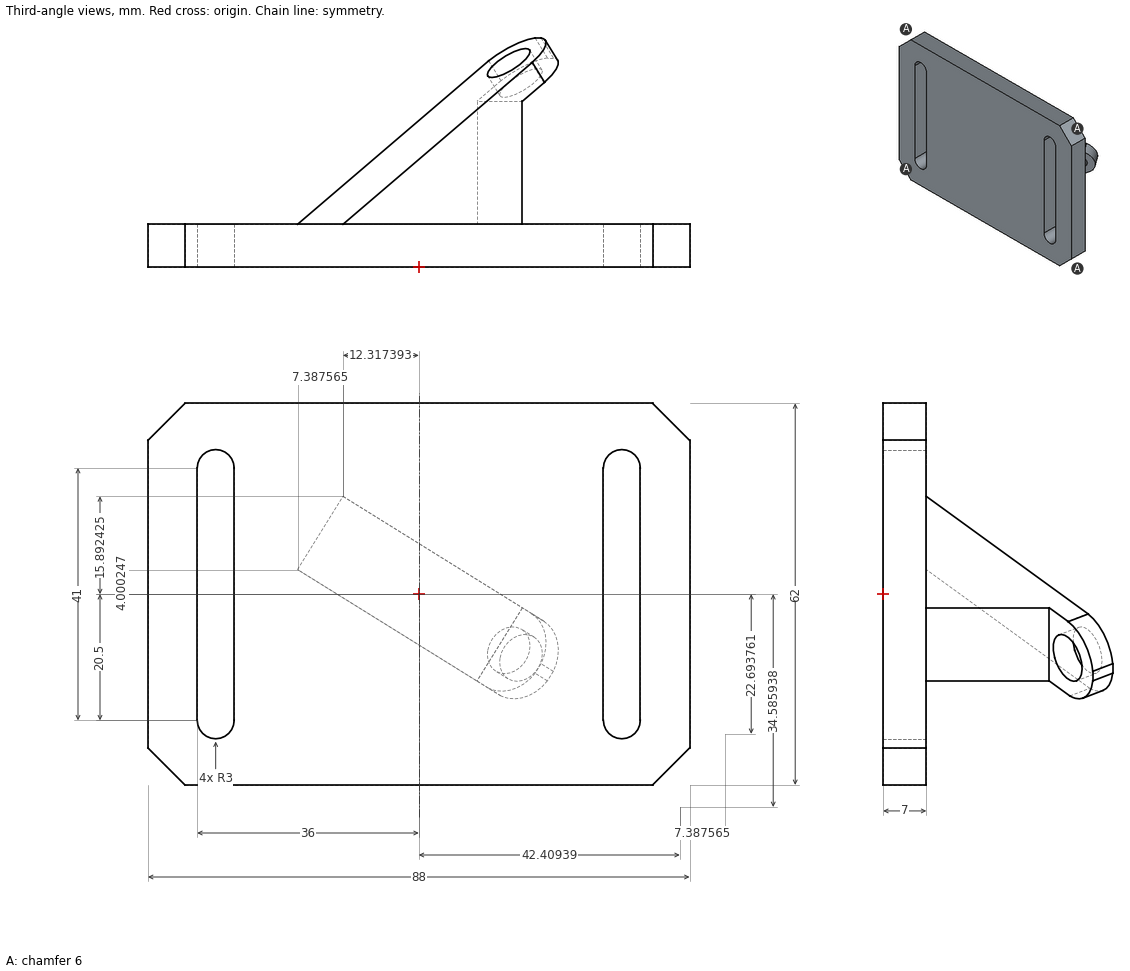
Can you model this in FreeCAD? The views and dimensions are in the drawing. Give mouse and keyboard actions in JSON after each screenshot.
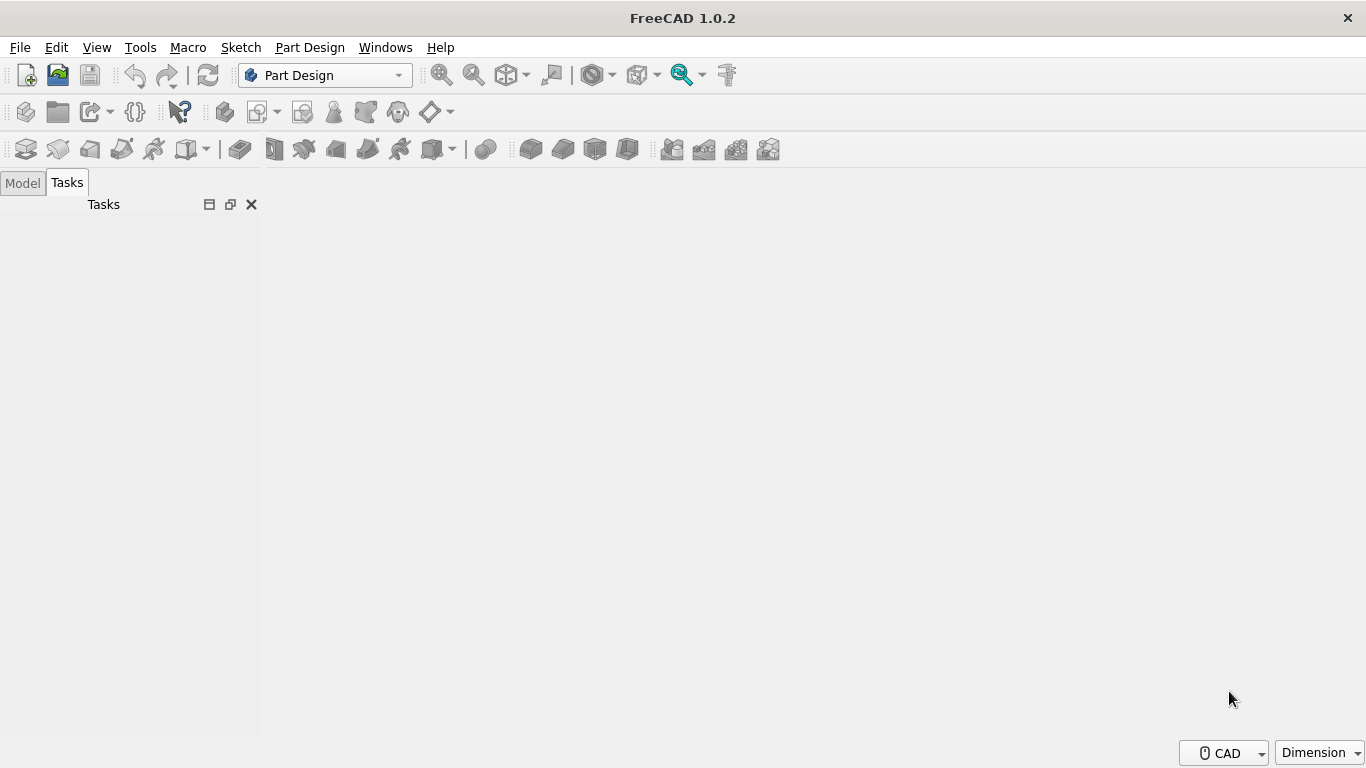
{"action": "left_click", "coordinate": [260, 76]}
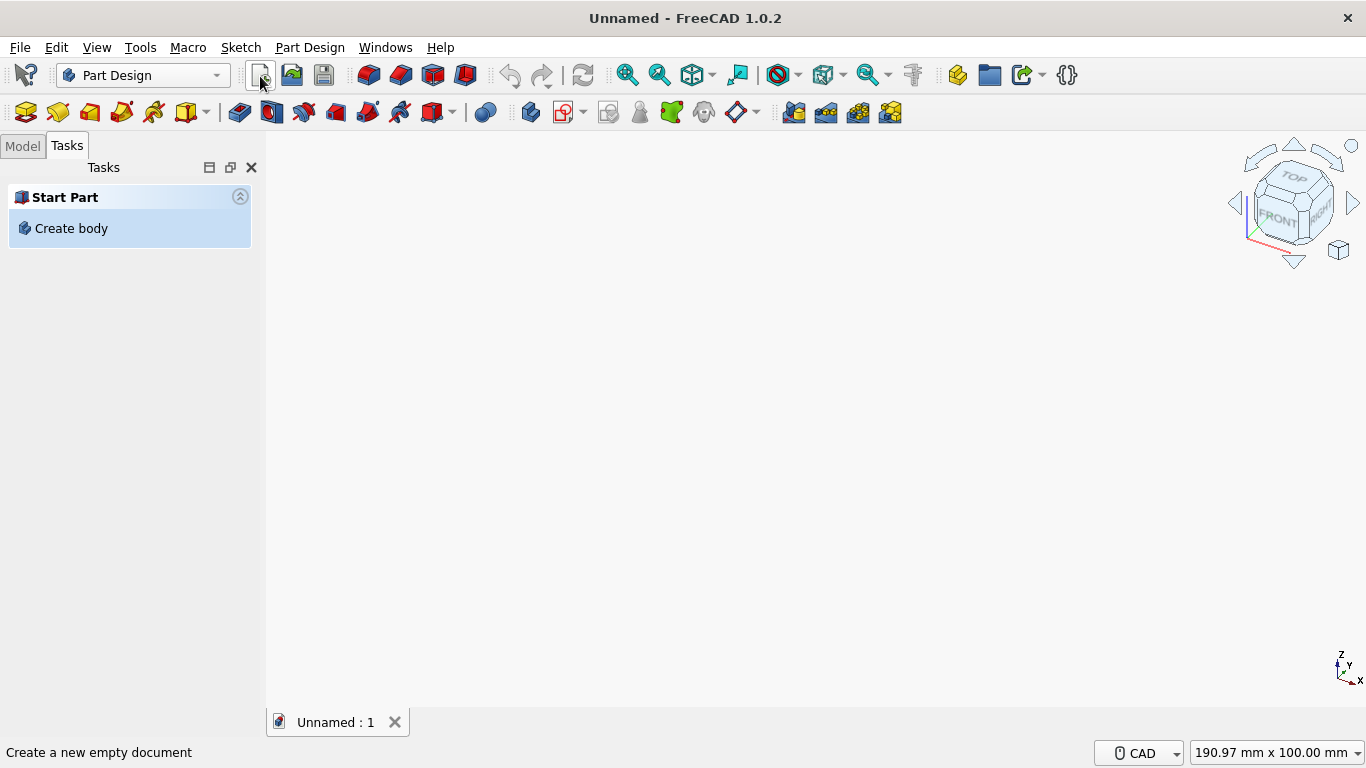
{"action": "left_click", "coordinate": [564, 112]}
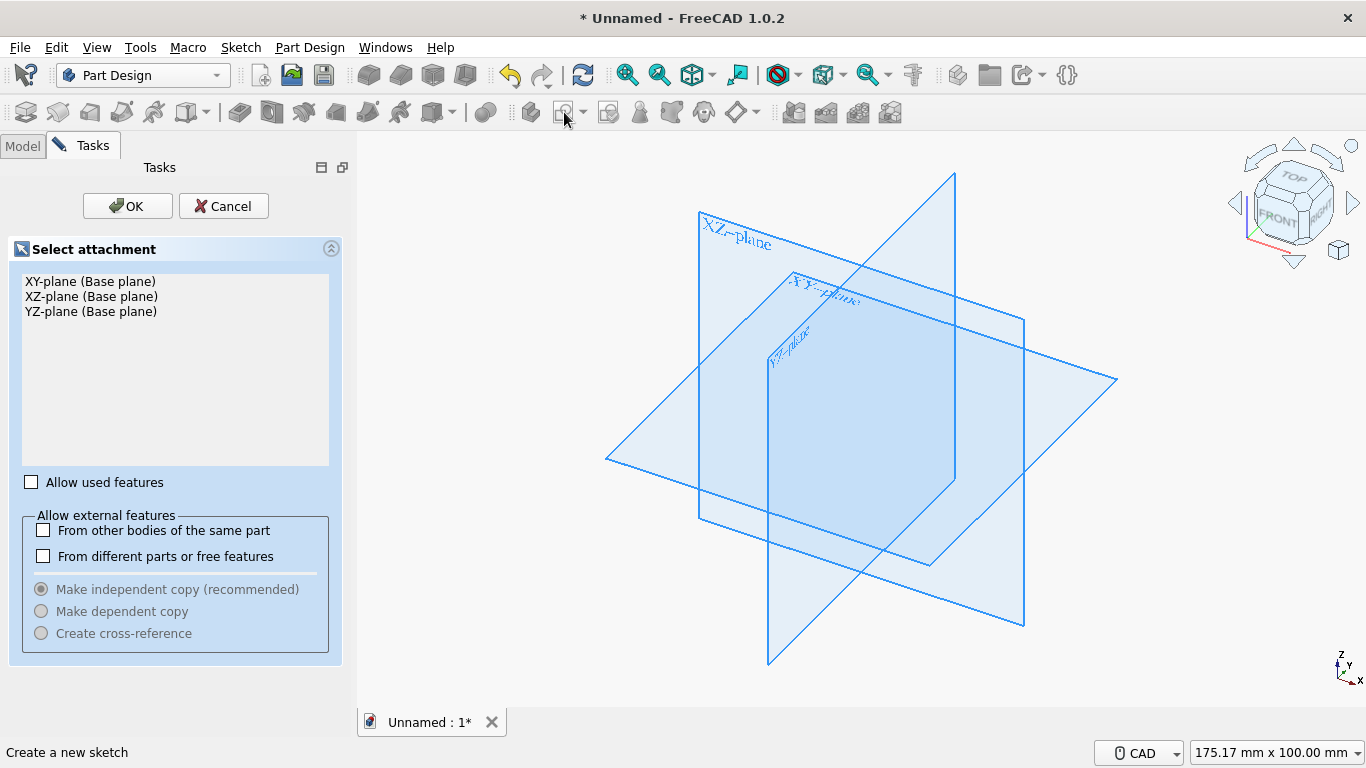
{"action": "left_click", "coordinate": [82, 296]}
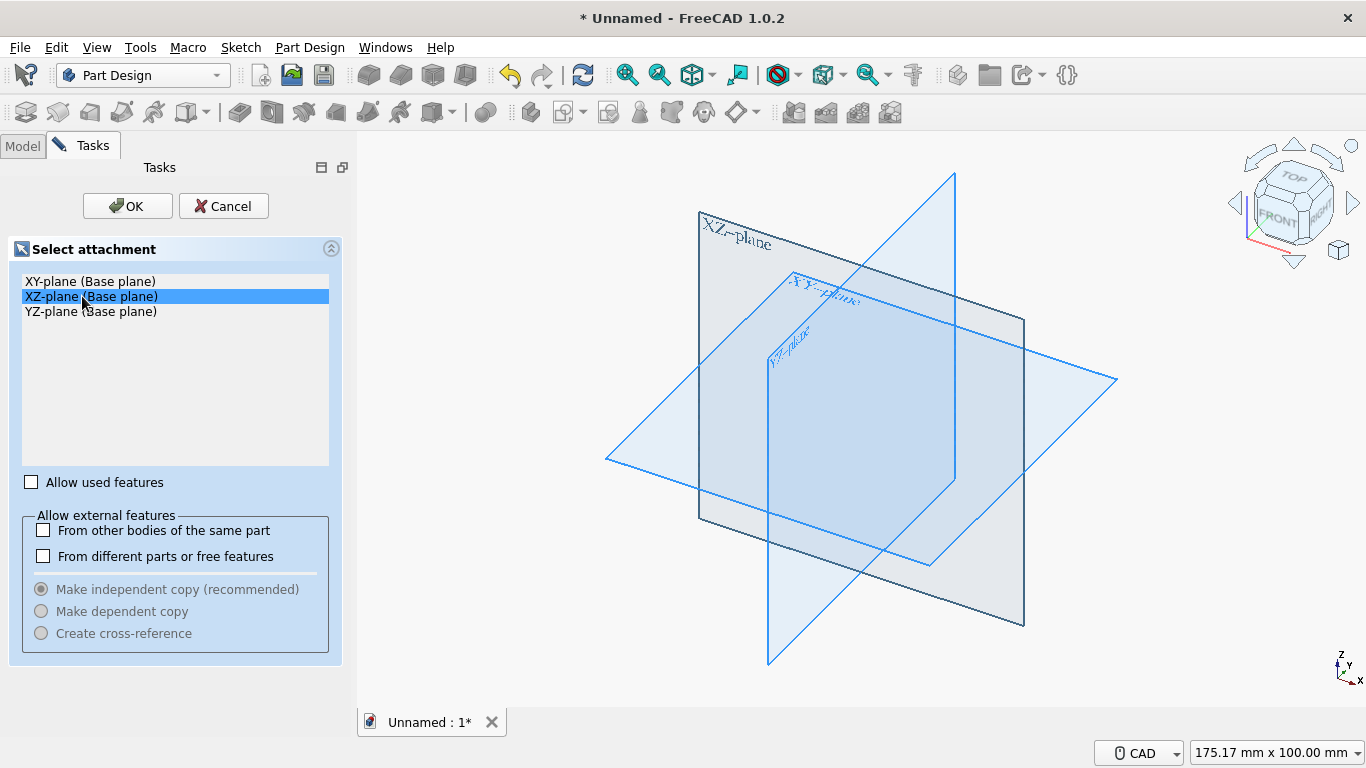
{"action": "left_click", "coordinate": [128, 206]}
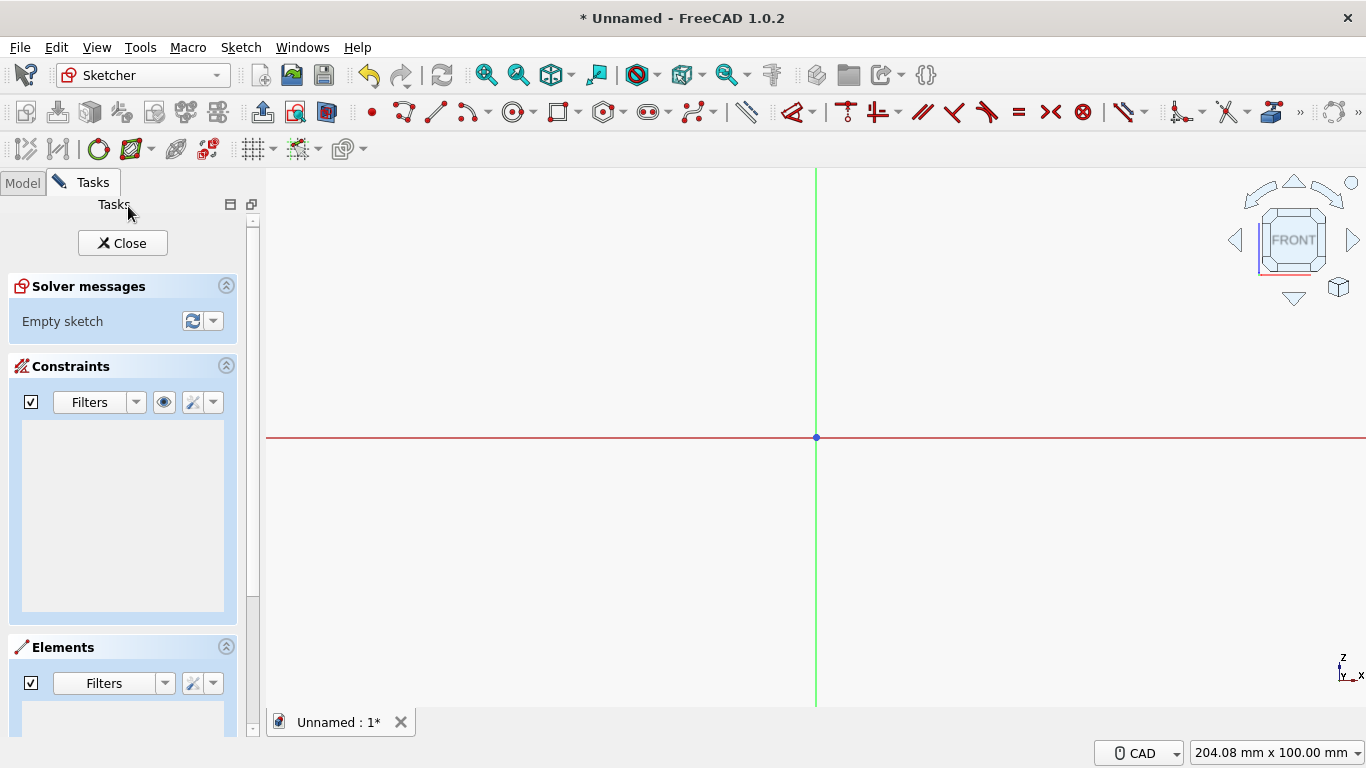
{"action": "left_click", "coordinate": [580, 112]}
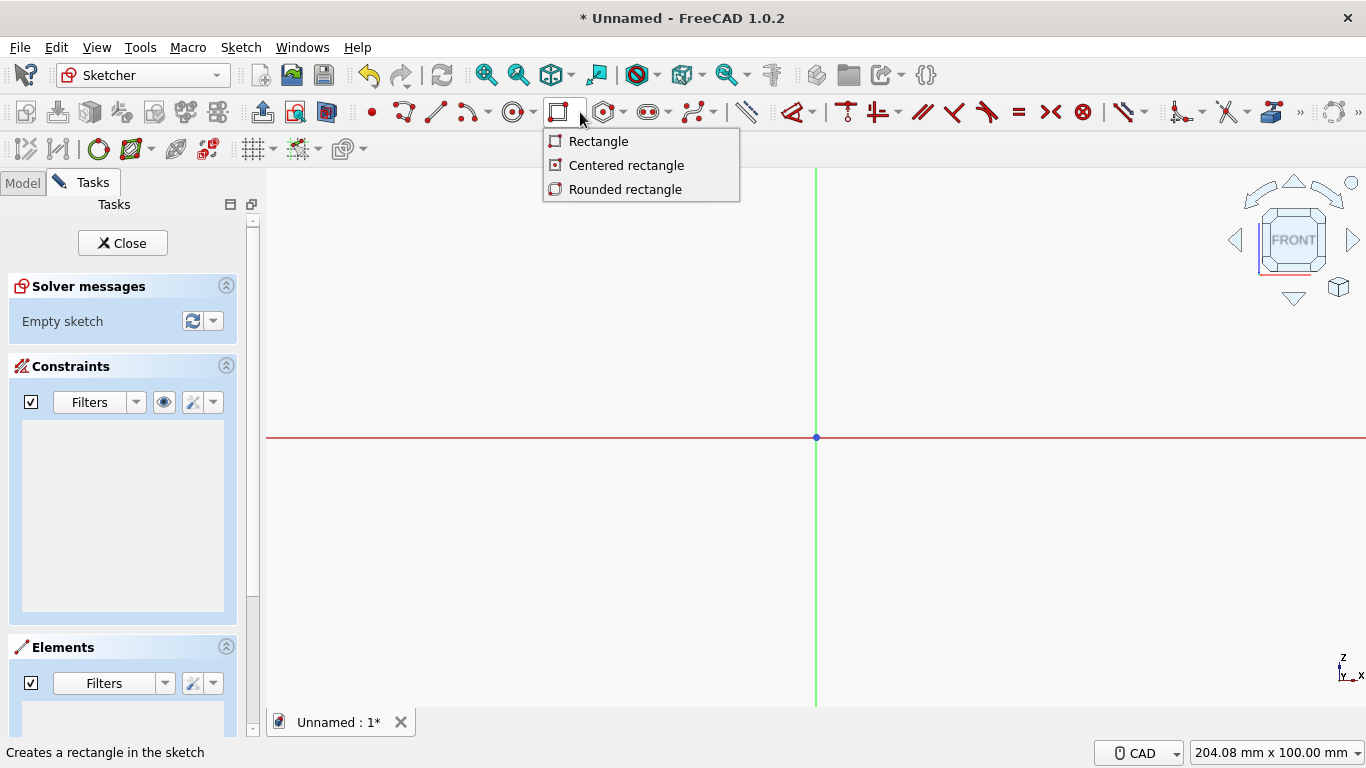
{"action": "left_click", "coordinate": [642, 165]}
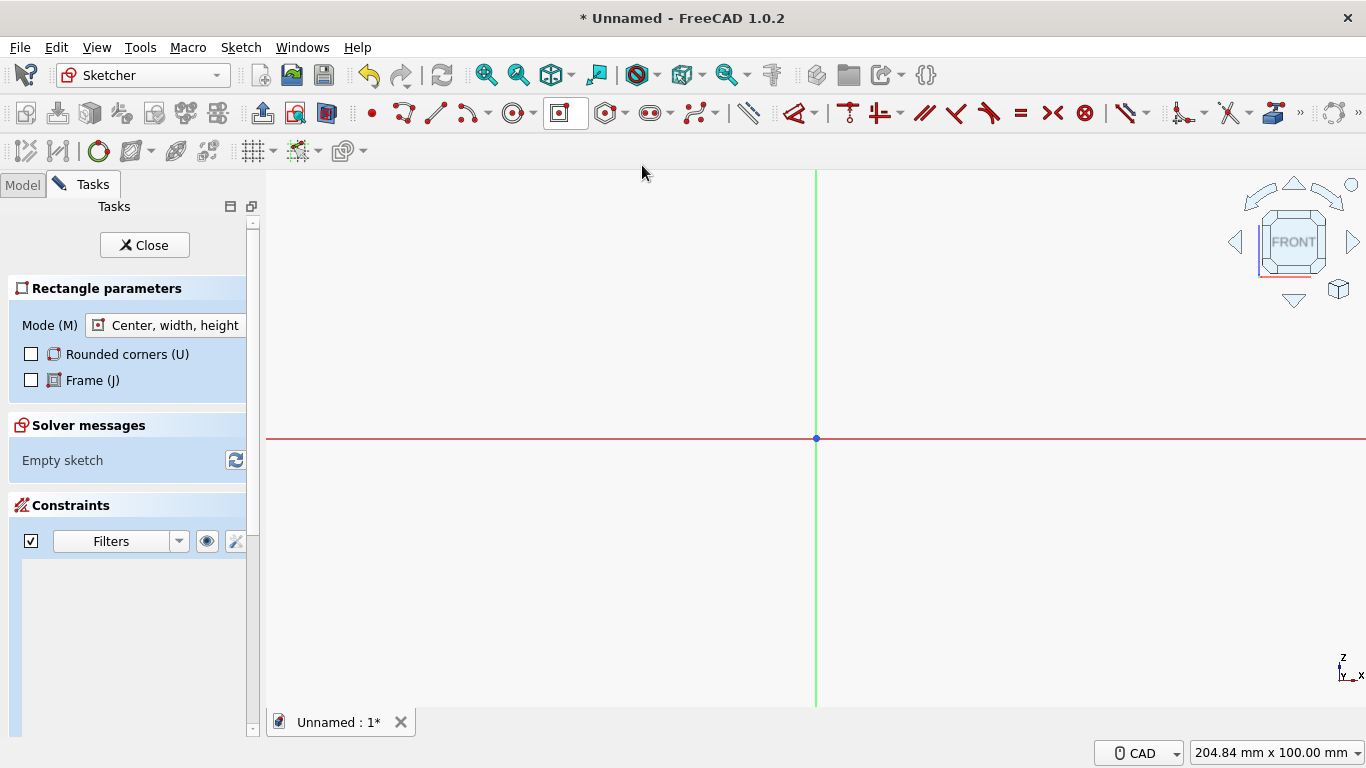
{"action": "left_click", "coordinate": [816, 438]}
{"action": "mouse_move", "coordinate": [1052, 272]}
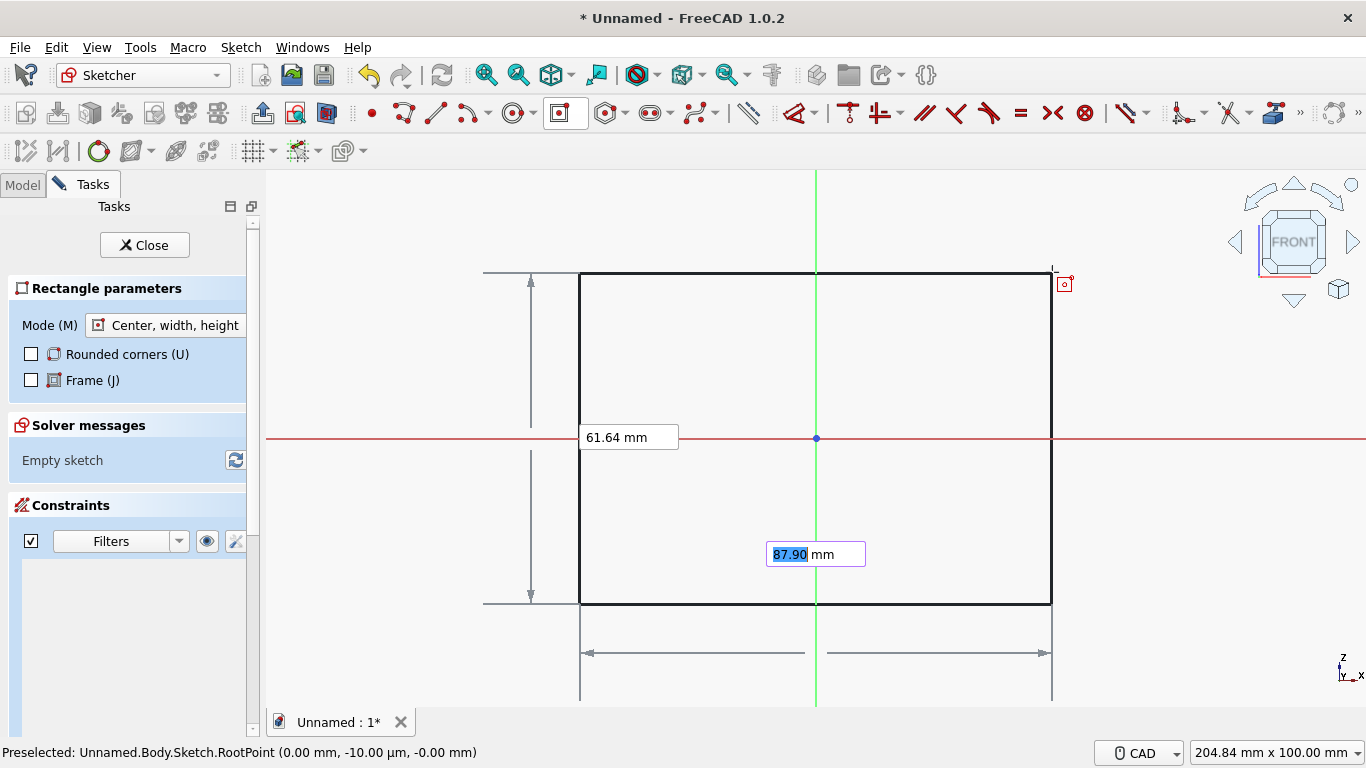
{"action": "type", "text": "88"}
{"action": "key", "text": "Tab"}
{"action": "type", "text": "62"}
{"action": "key", "text": "Return"}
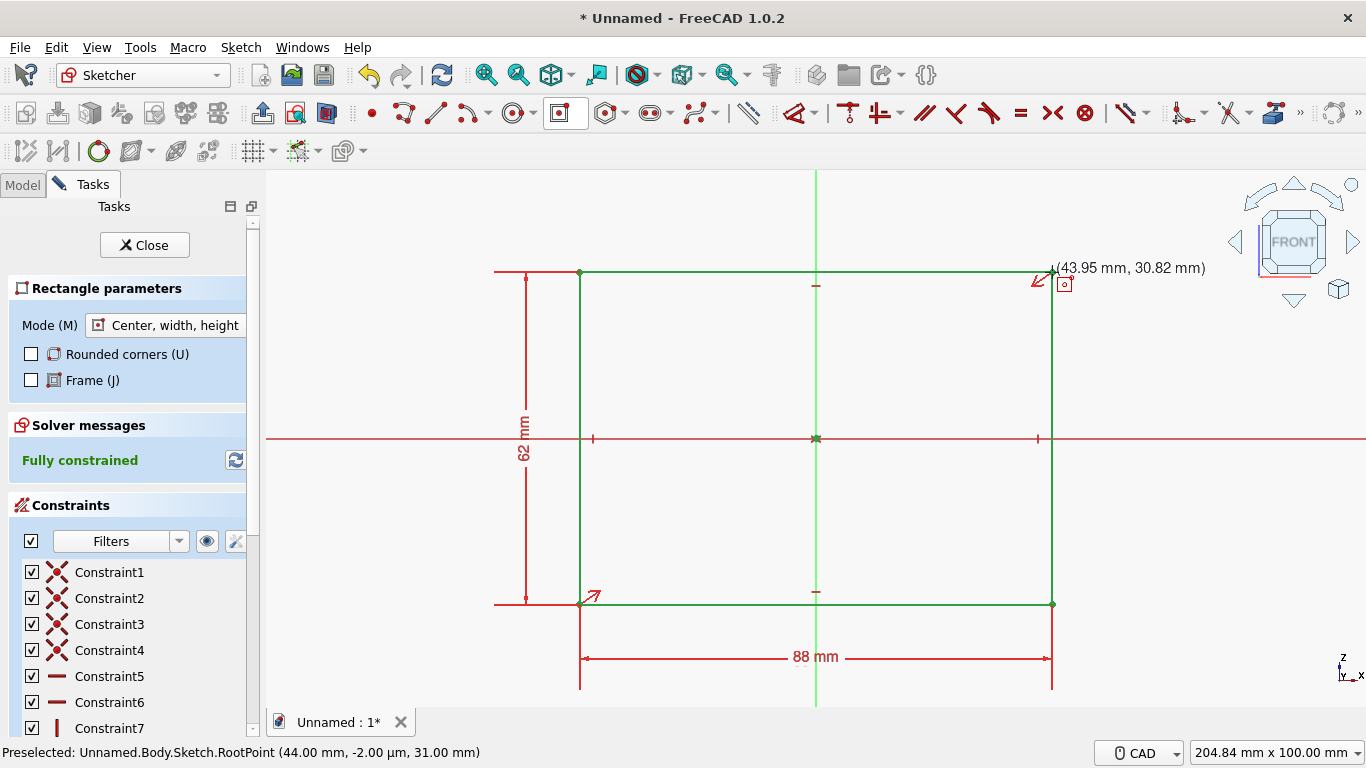
{"action": "left_click", "coordinate": [650, 114]}